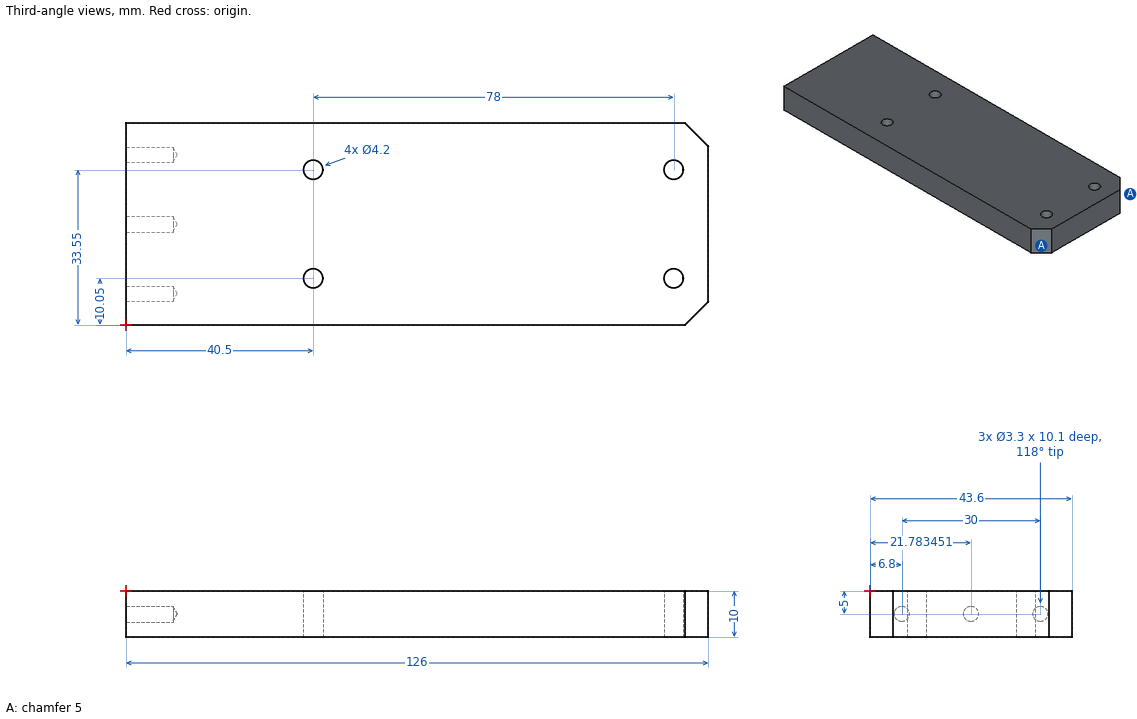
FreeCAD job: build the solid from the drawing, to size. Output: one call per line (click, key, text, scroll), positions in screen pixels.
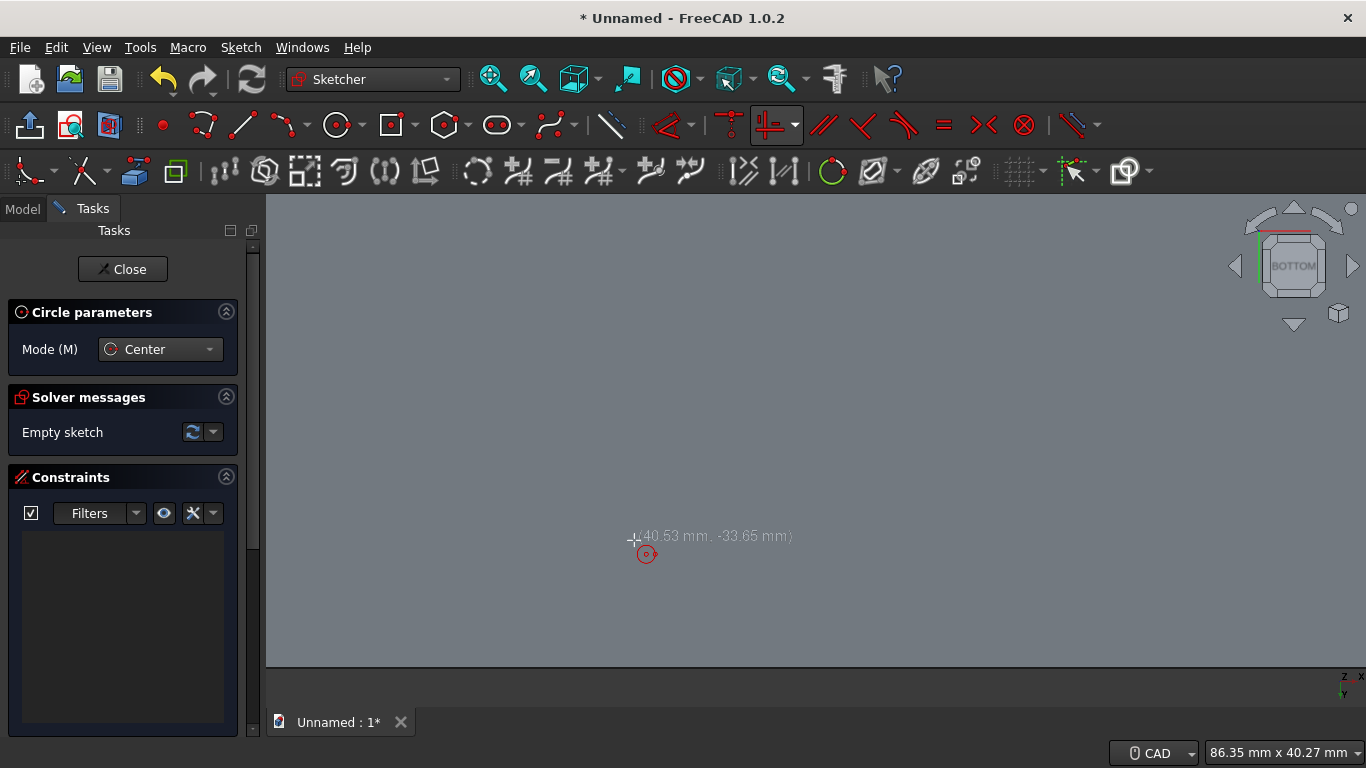
click(633, 540)
move(652, 521)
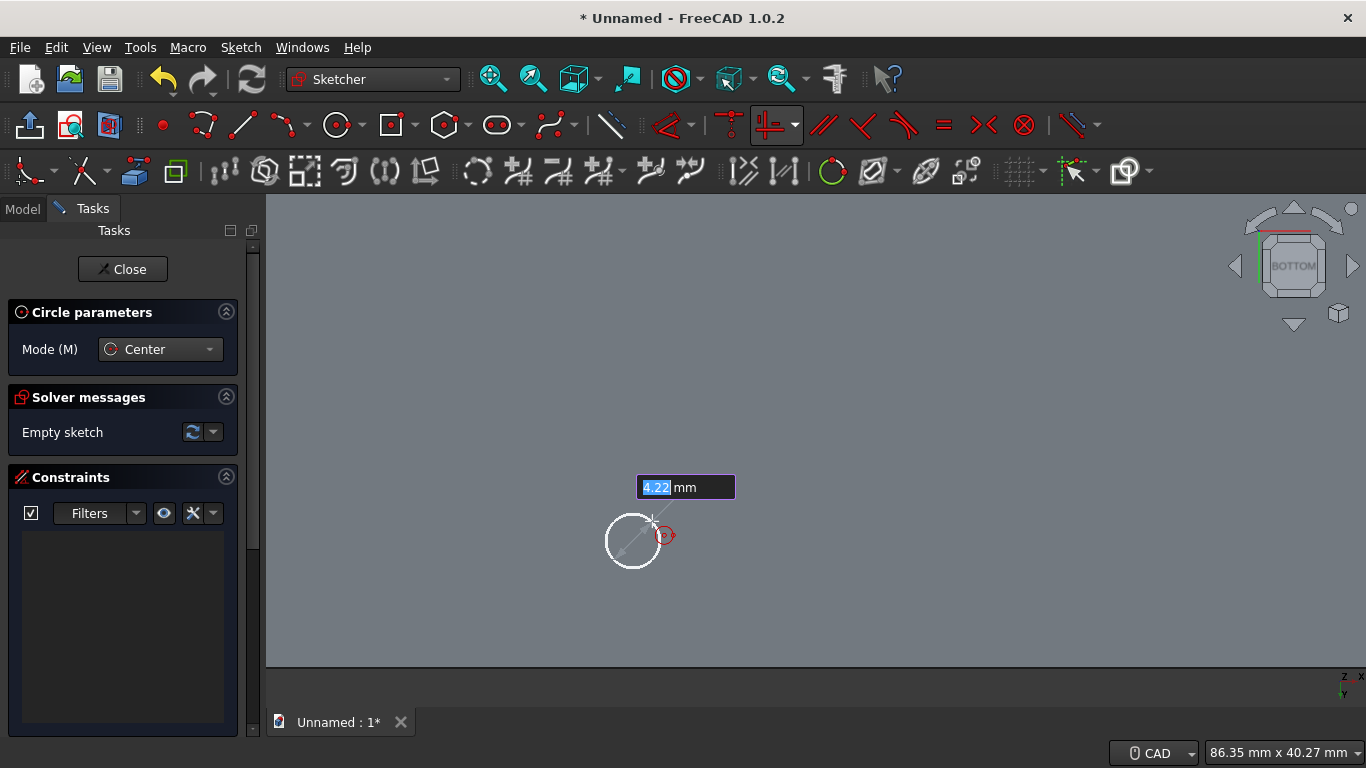
text(4.2)
key(Return)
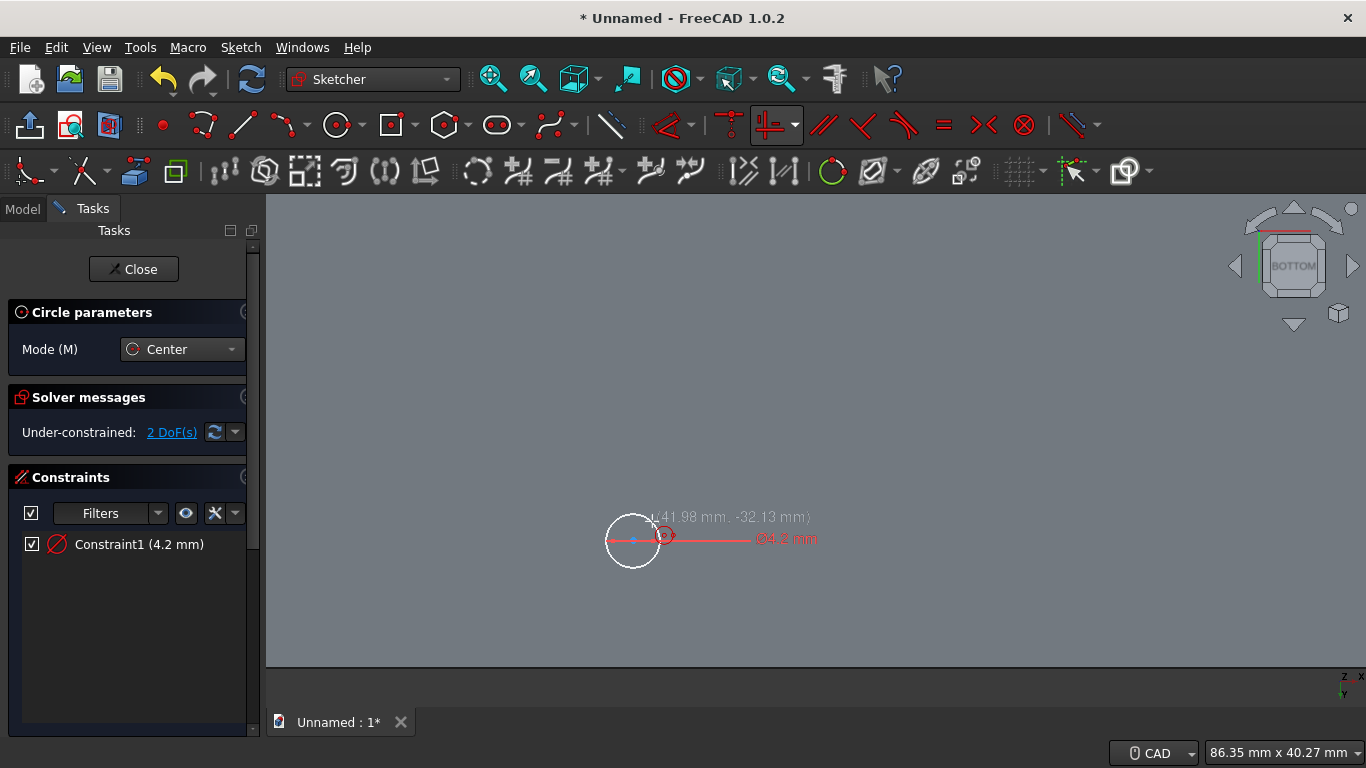
click(633, 241)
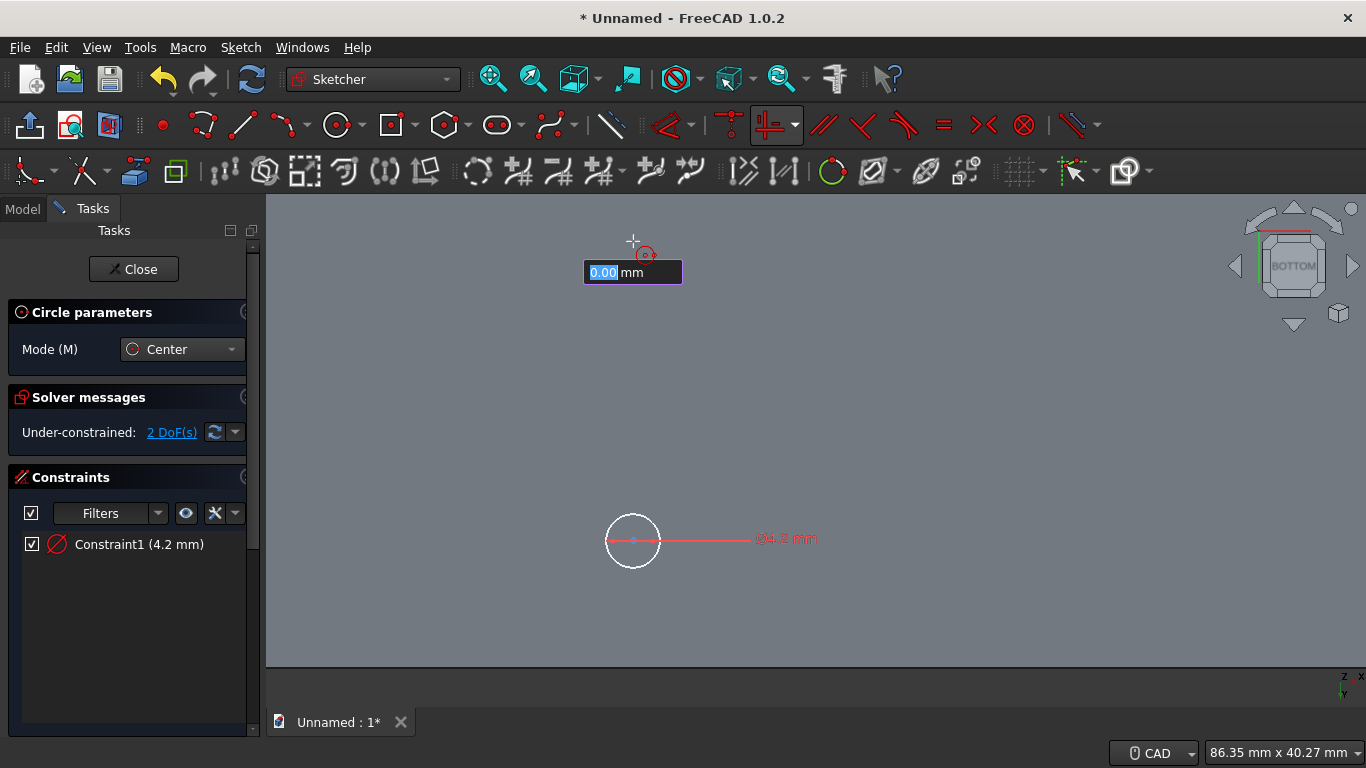
scroll(635, 541, down, 4)
move(643, 398)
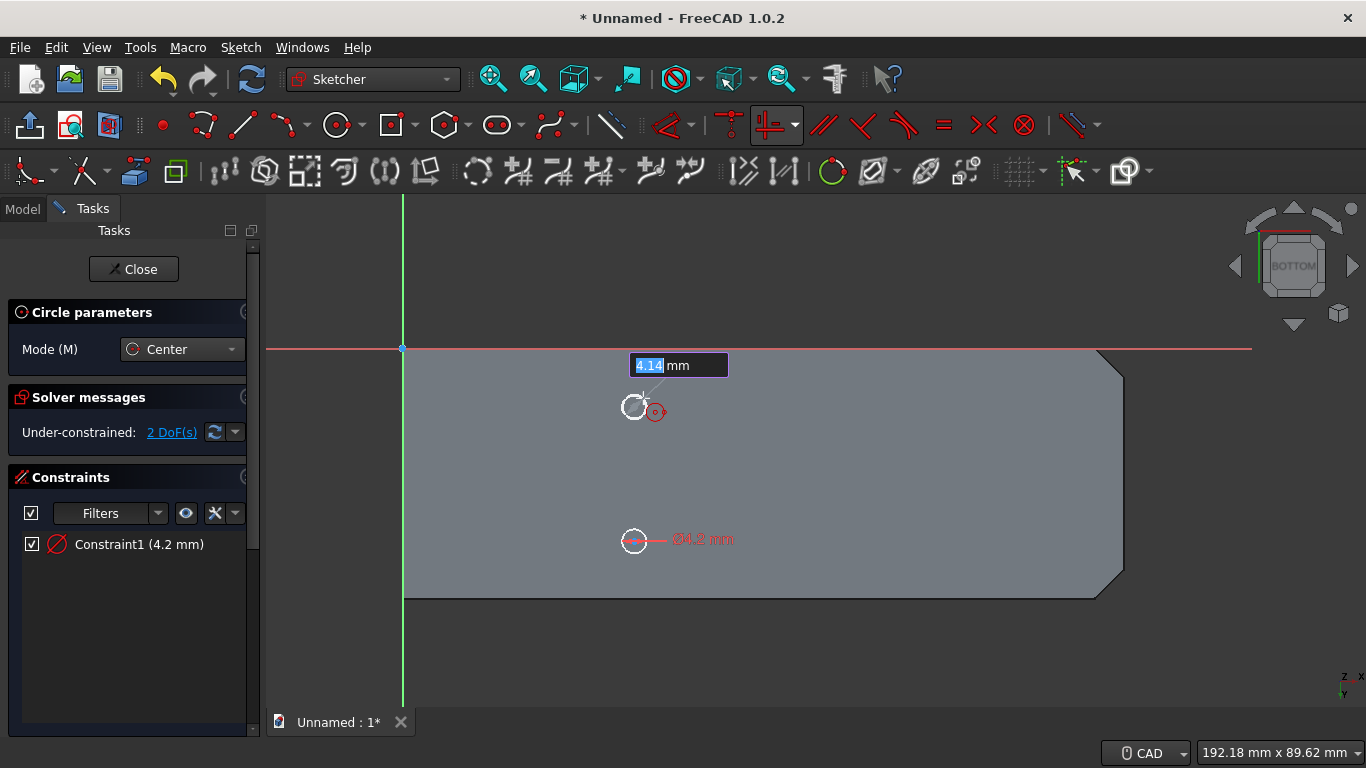
text(4.2)
key(Return)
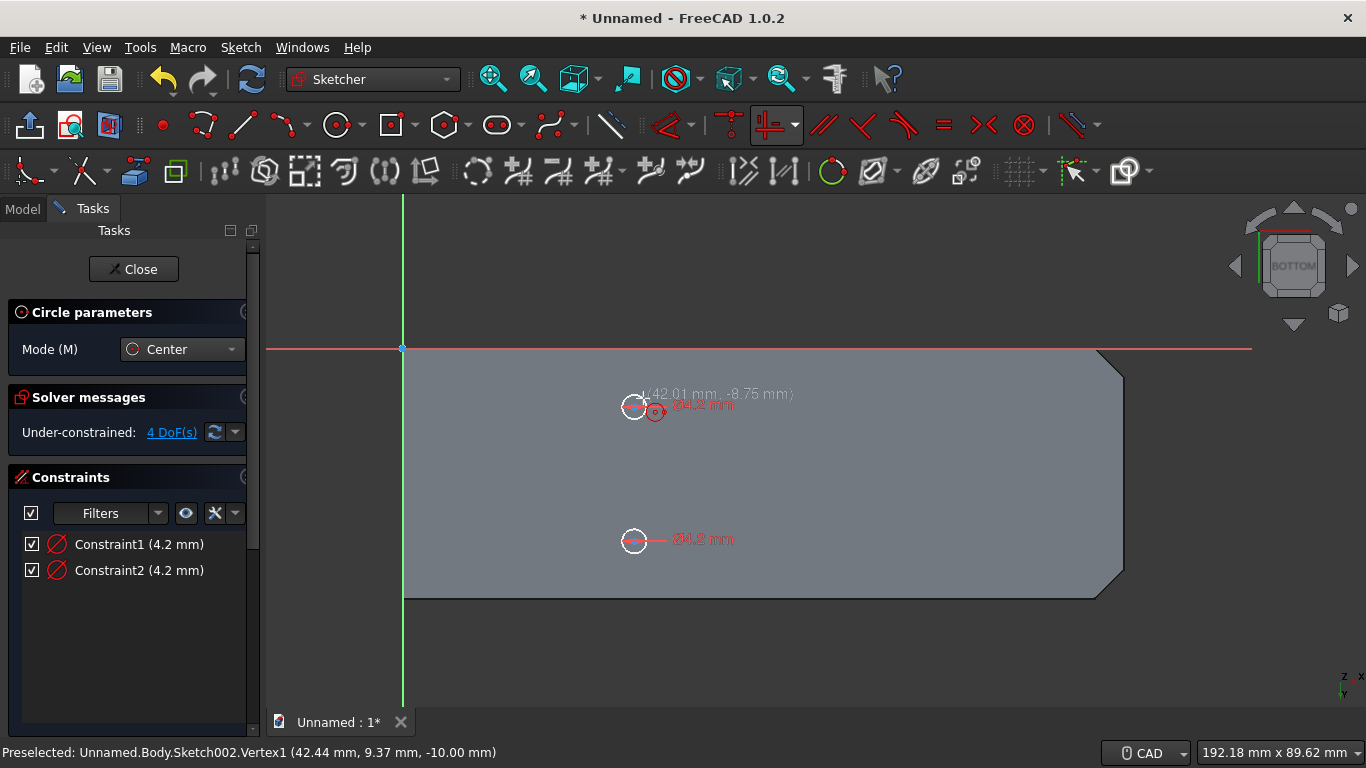
scroll(1081, 541, up, 4)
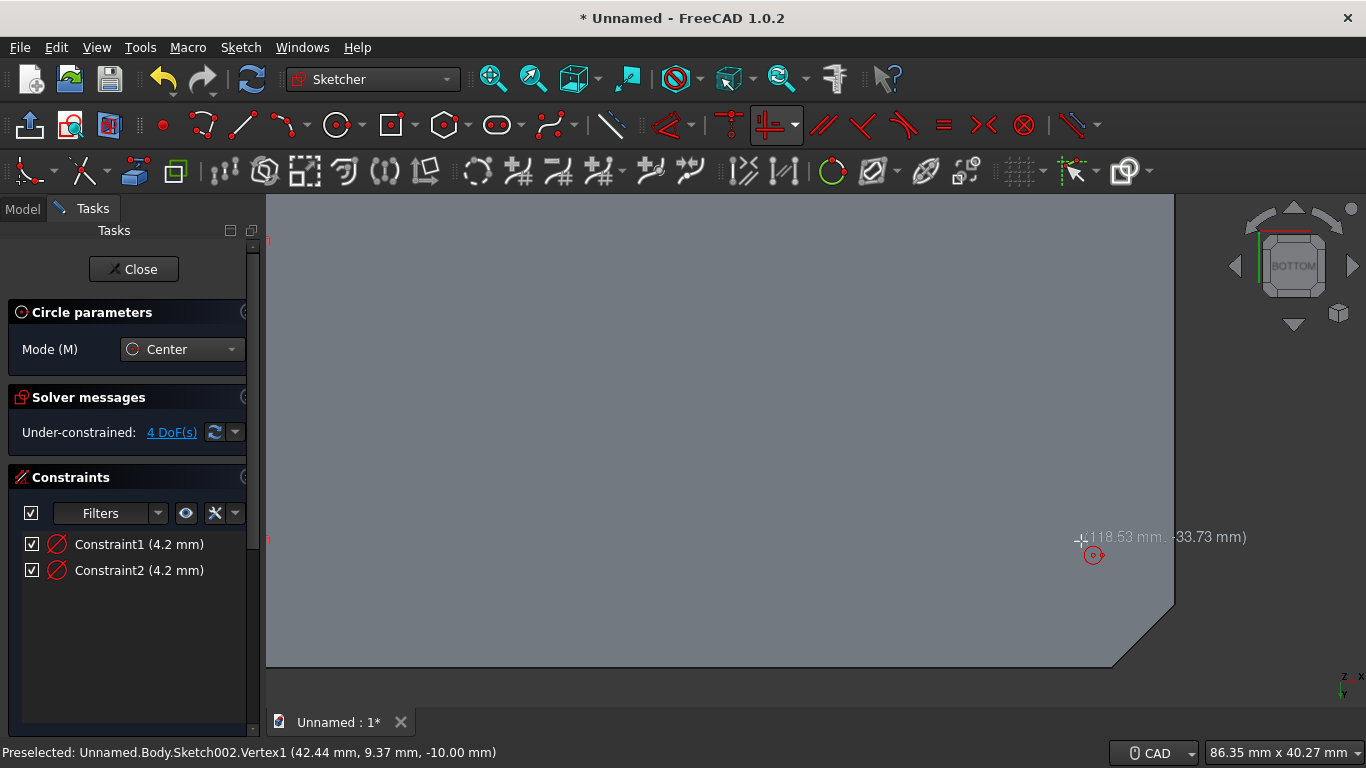
click(1080, 540)
move(1099, 521)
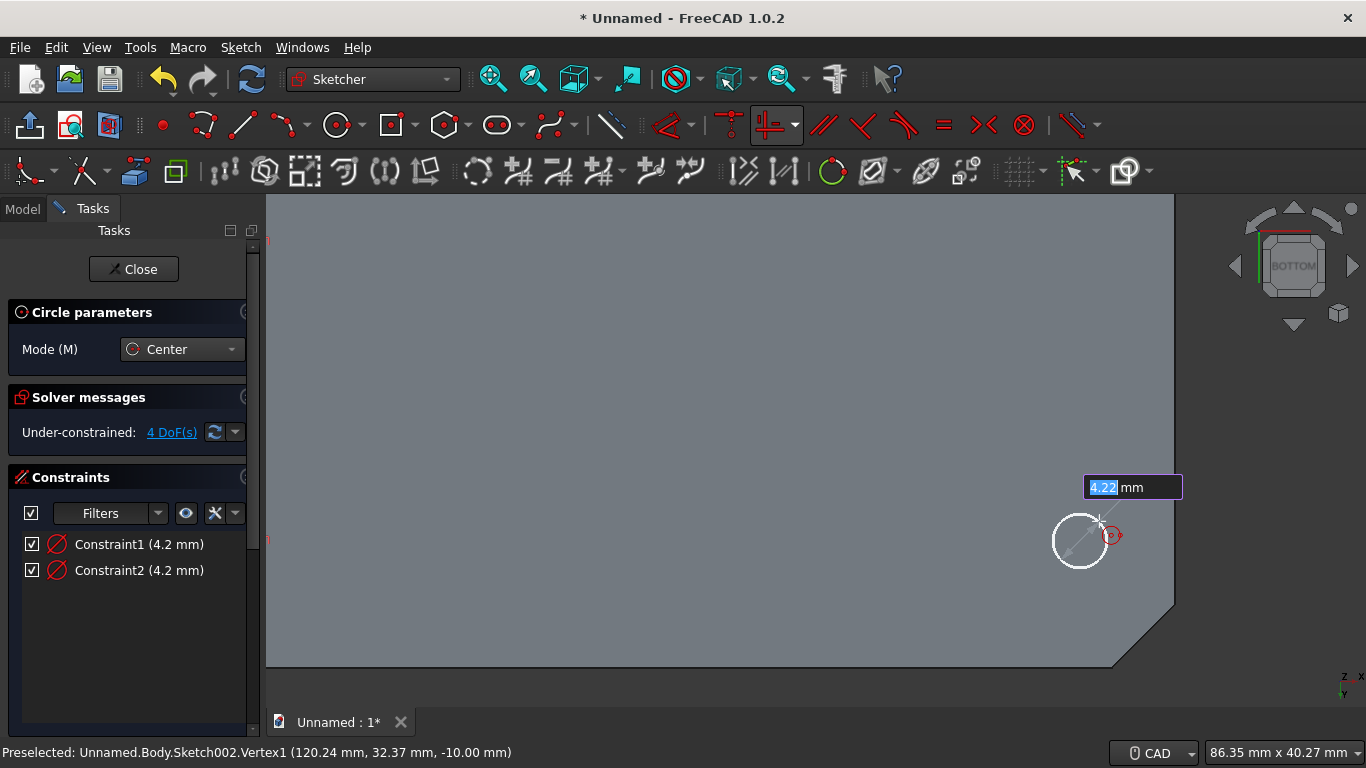
text(4.2)
key(Return)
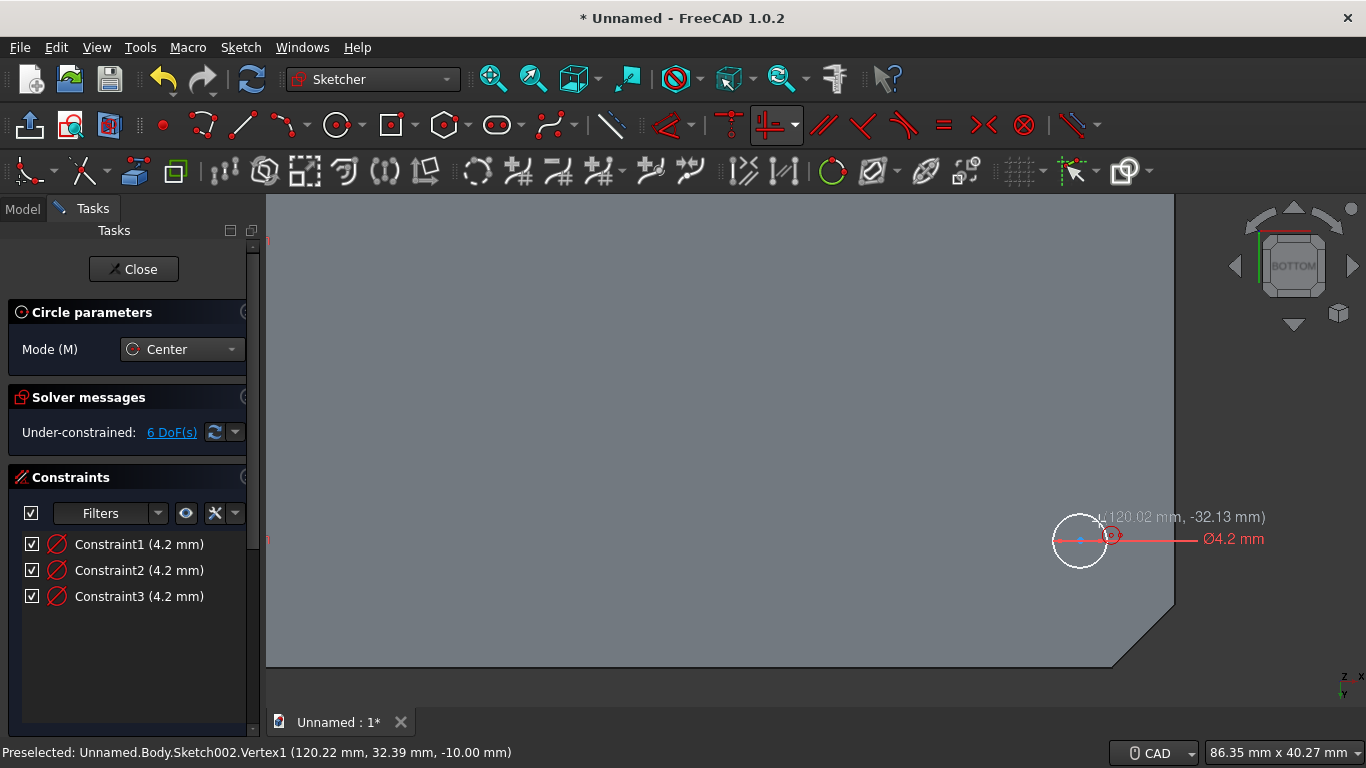
click(1080, 241)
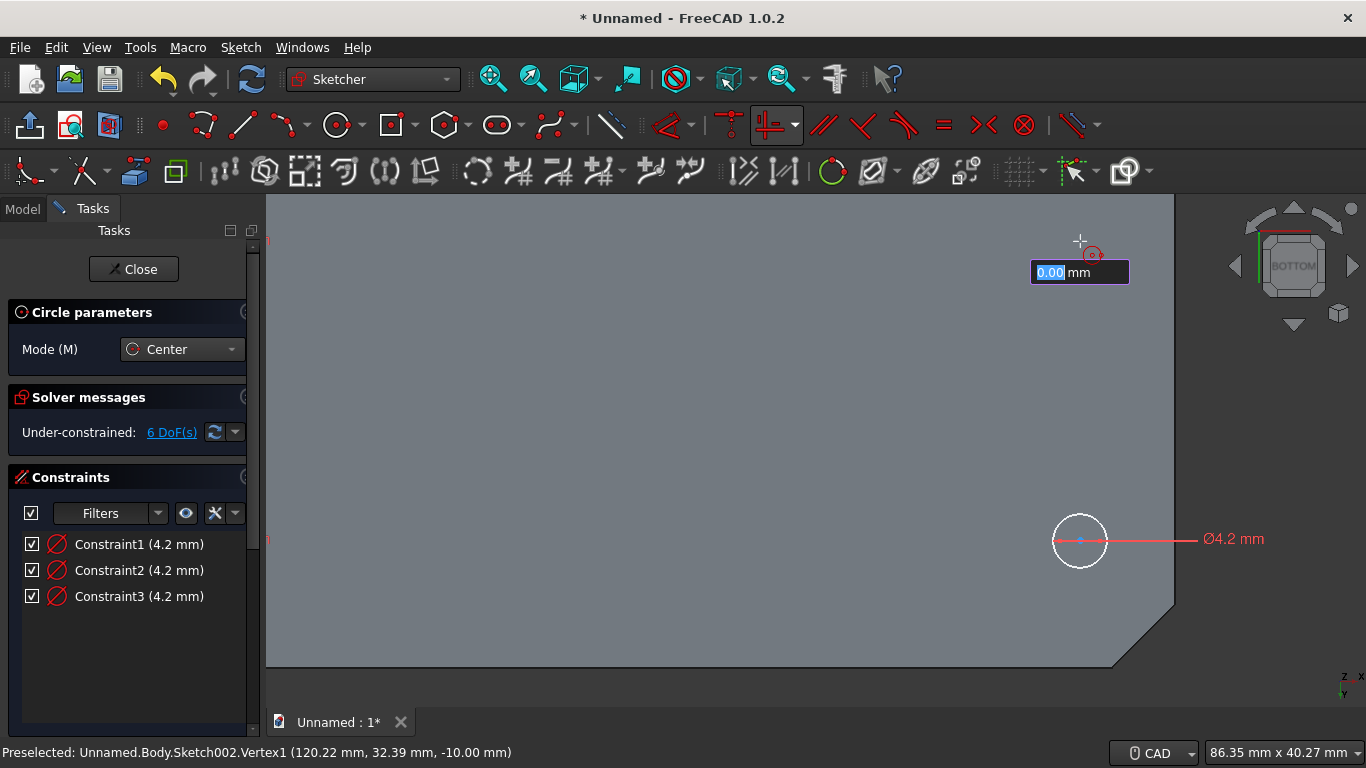
scroll(1081, 541, down, 4)
move(1089, 398)